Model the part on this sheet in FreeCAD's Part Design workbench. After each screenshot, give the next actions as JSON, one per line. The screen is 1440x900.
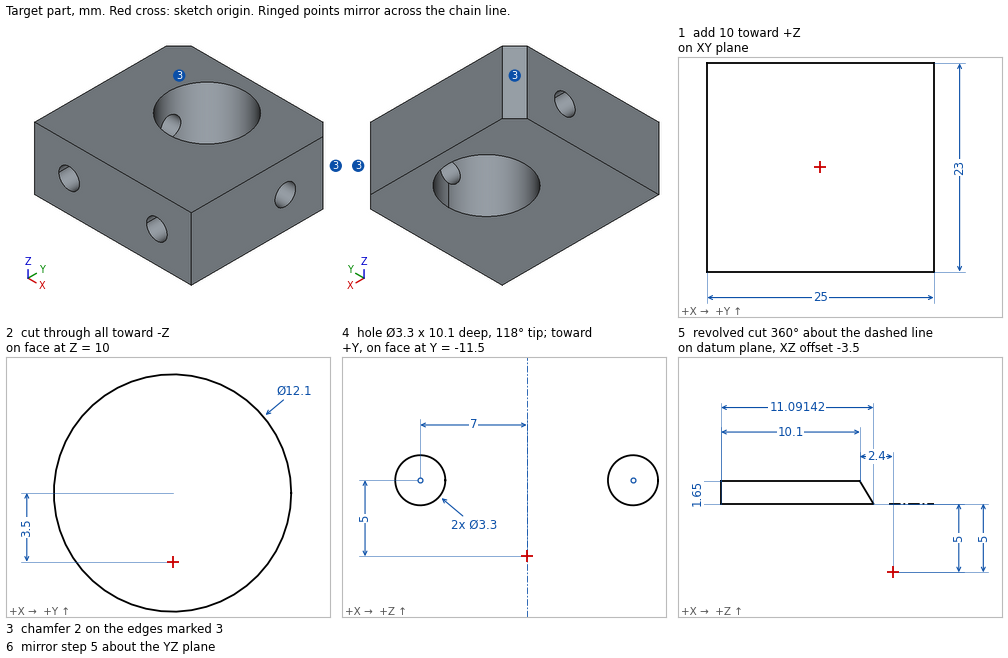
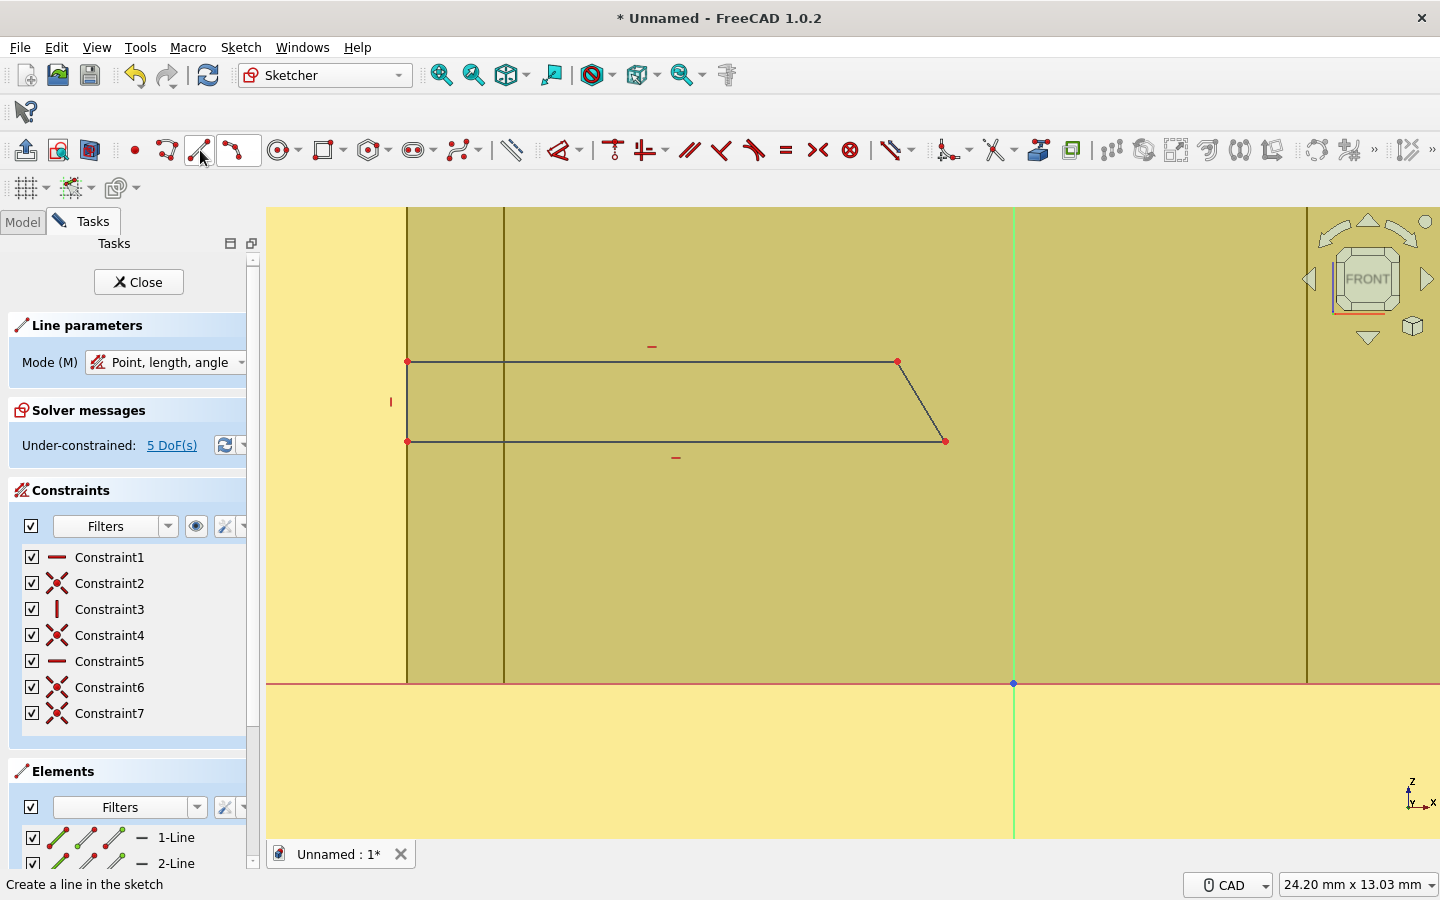
{"action": "left_click", "coordinate": [999, 441]}
{"action": "left_click", "coordinate": [1161, 441]}
{"action": "key", "text": "Escape"}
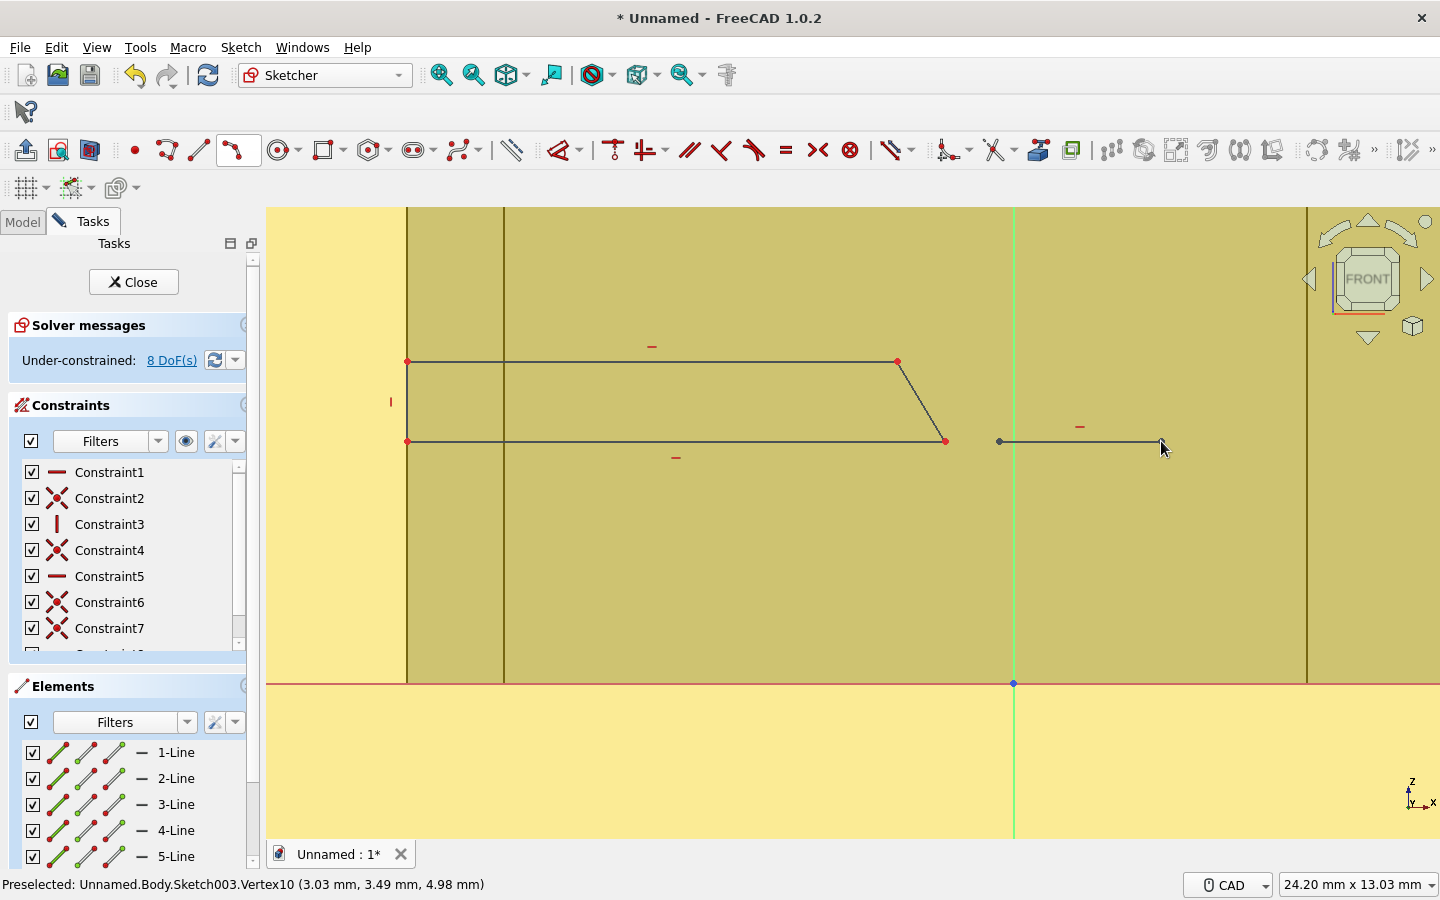
{"action": "left_click", "coordinate": [1048, 442]}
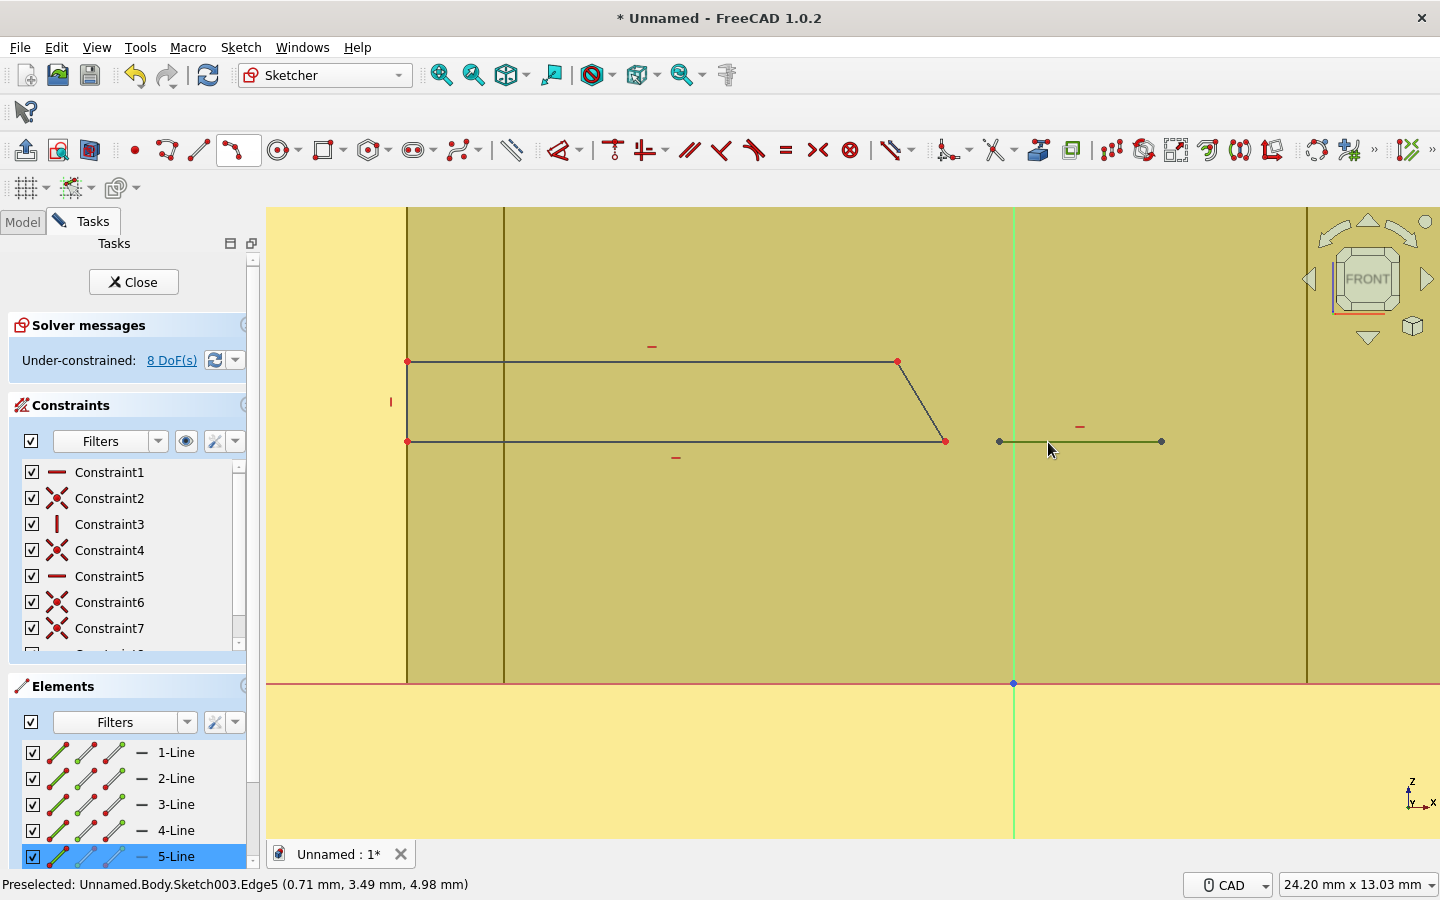
{"action": "key", "text": "g n"}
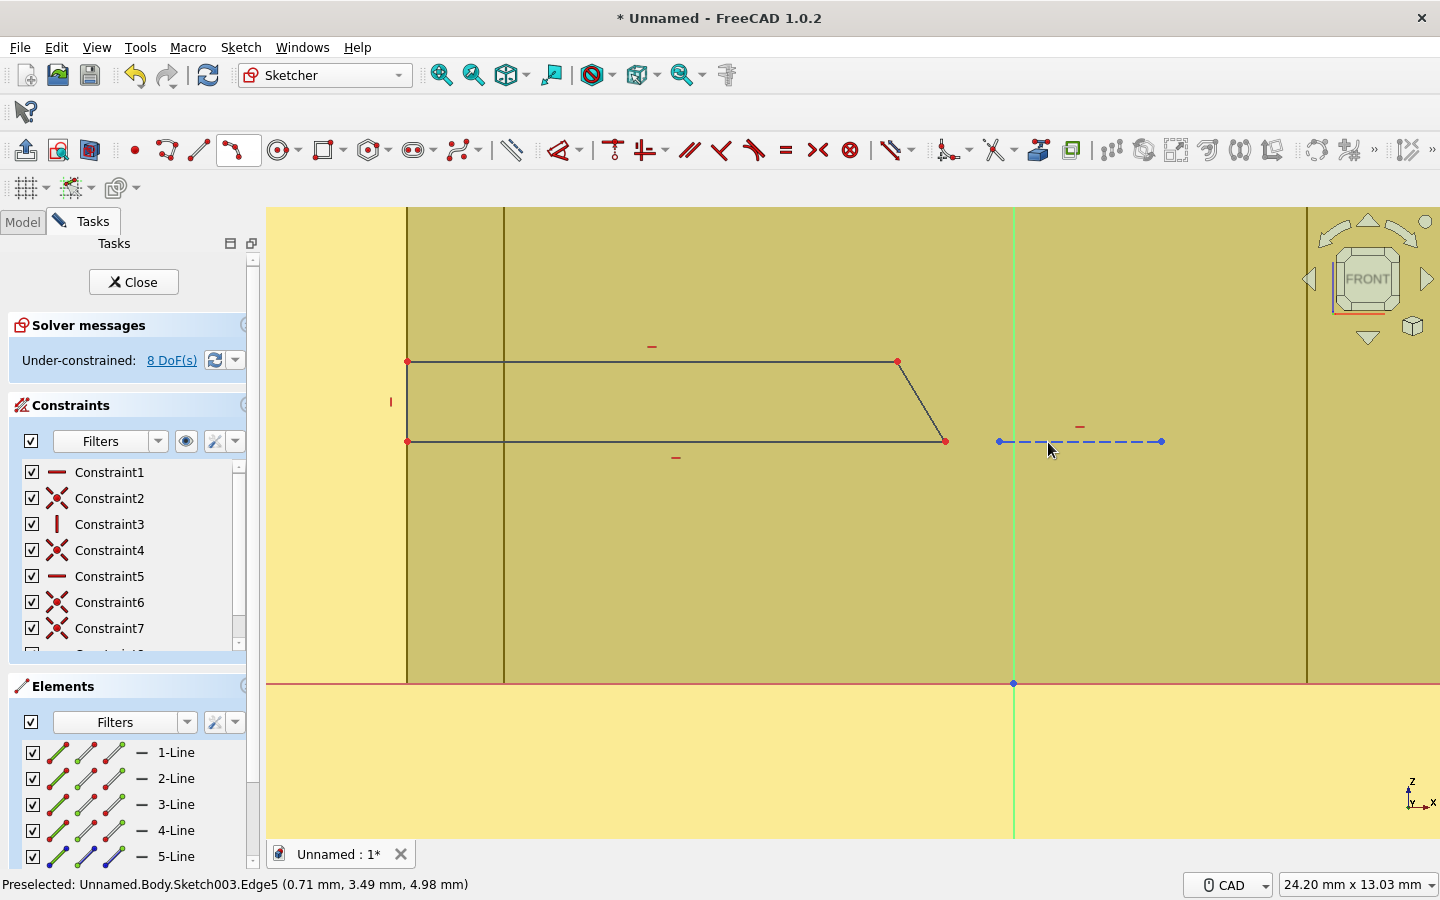
{"action": "left_click", "coordinate": [558, 150]}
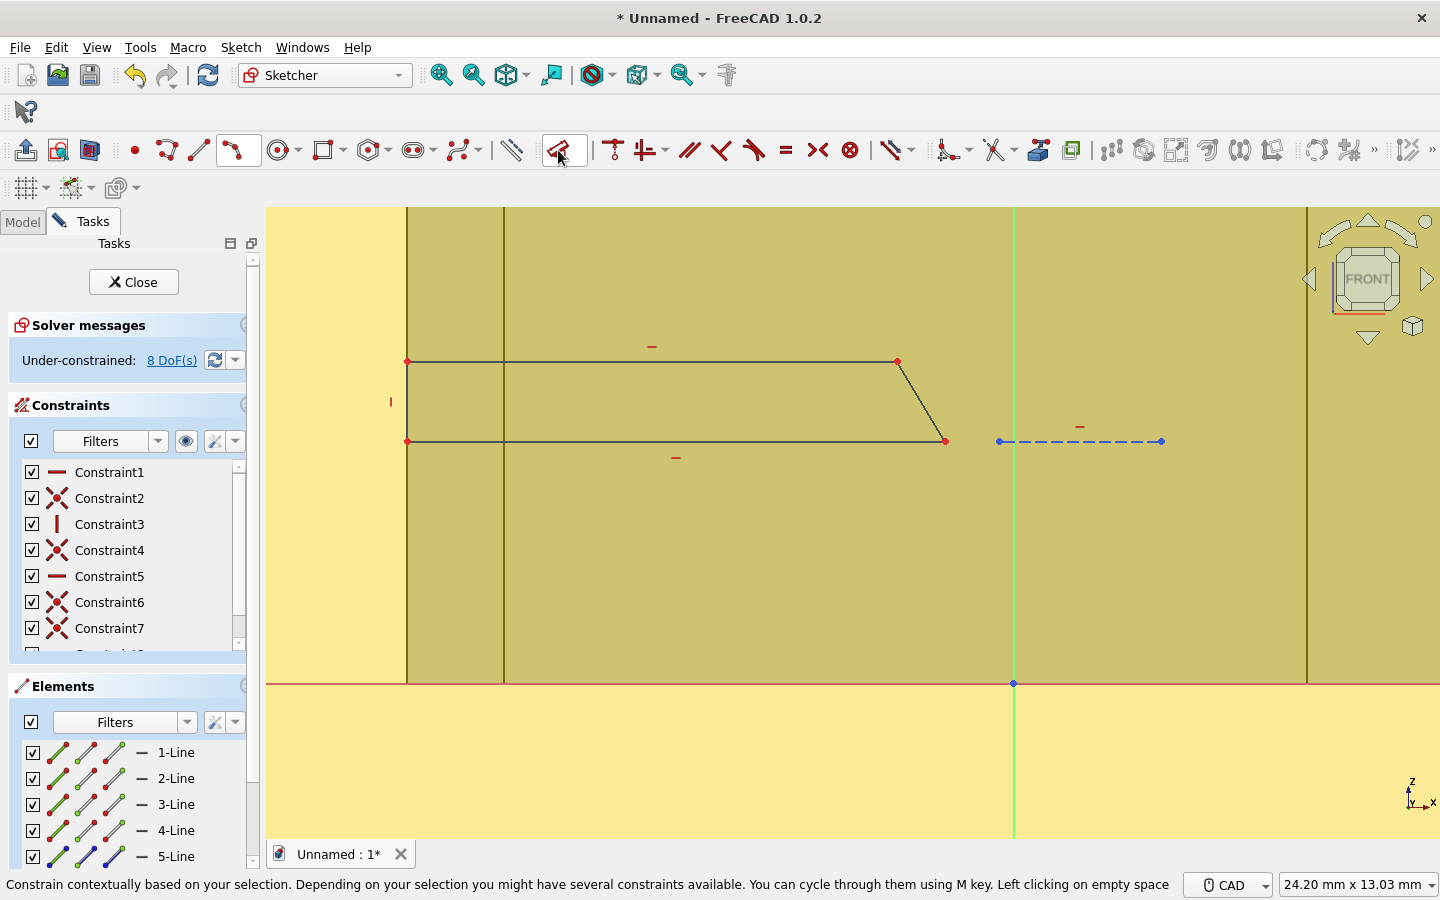
{"action": "left_click", "coordinate": [945, 442]}
{"action": "left_click", "coordinate": [1048, 563]}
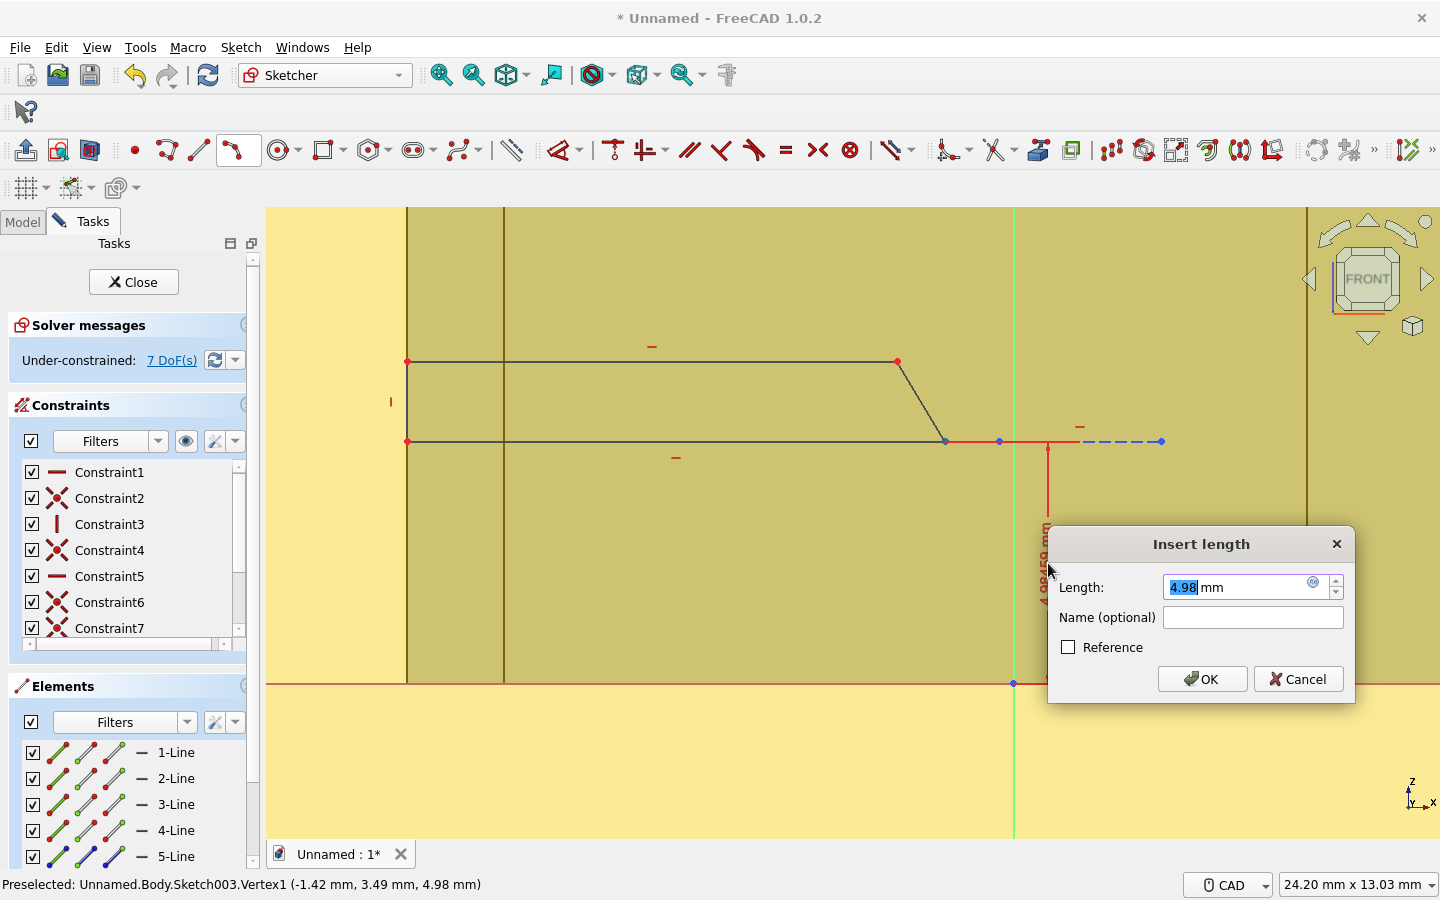
{"action": "type", "text": "5"}
{"action": "key", "text": "Return"}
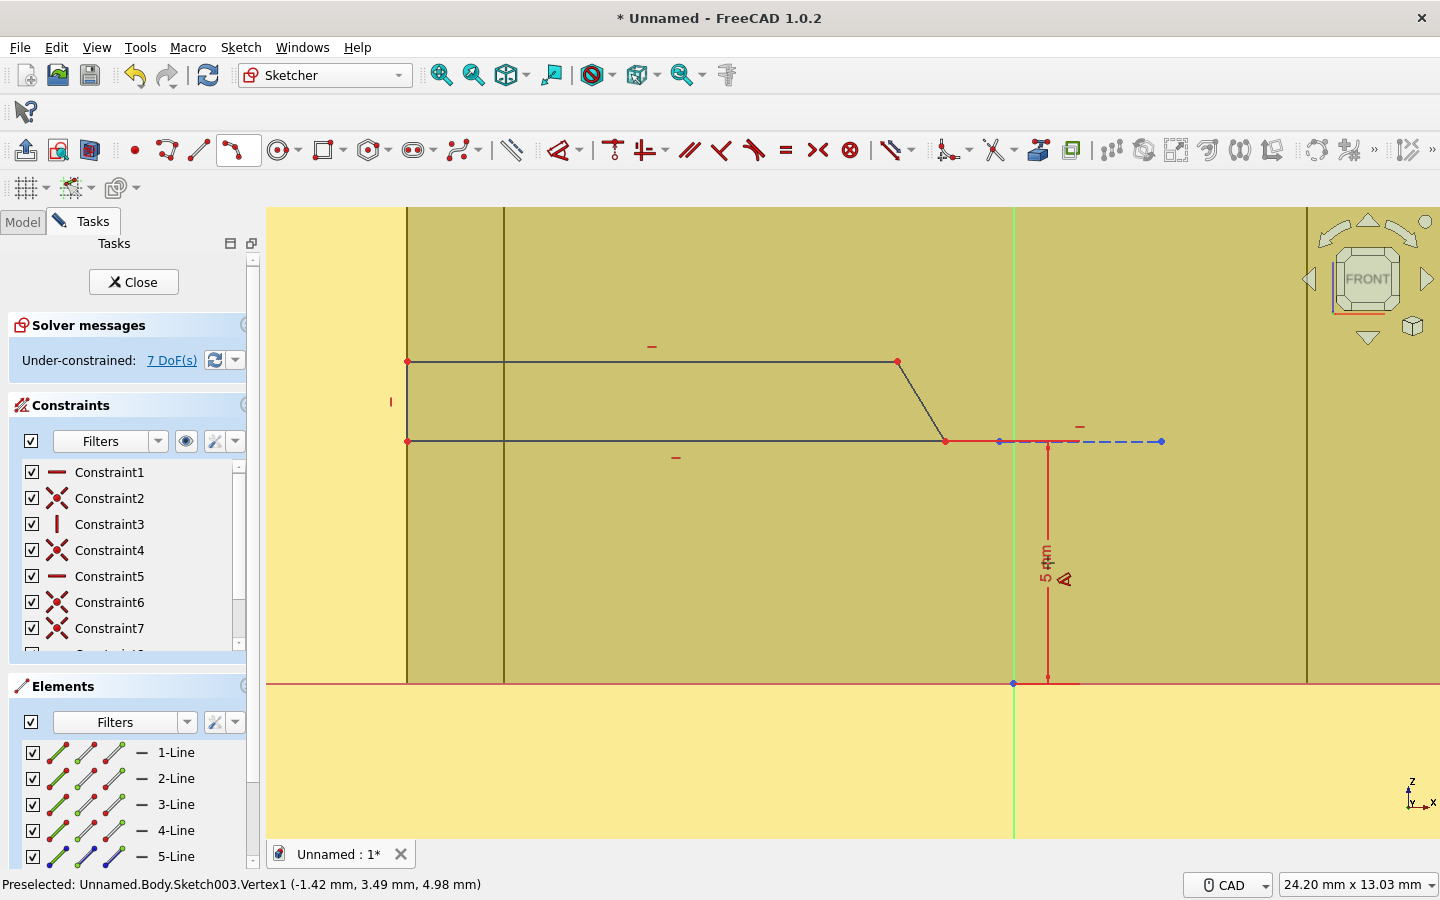
{"action": "left_click", "coordinate": [999, 442]}
{"action": "left_click", "coordinate": [1048, 507]}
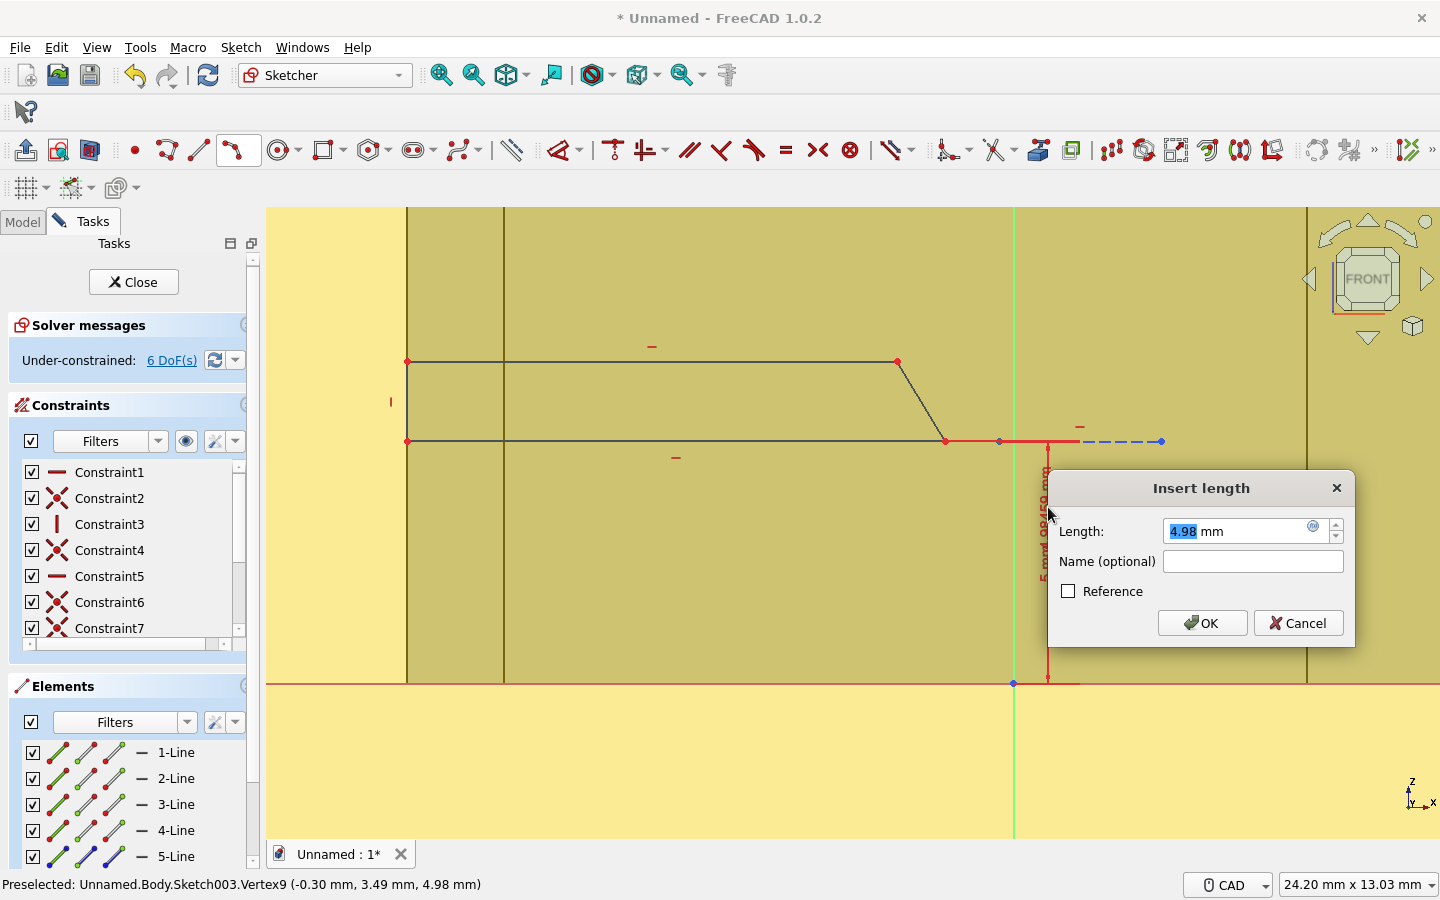
{"action": "type", "text": "5"}
{"action": "key", "text": "Return"}